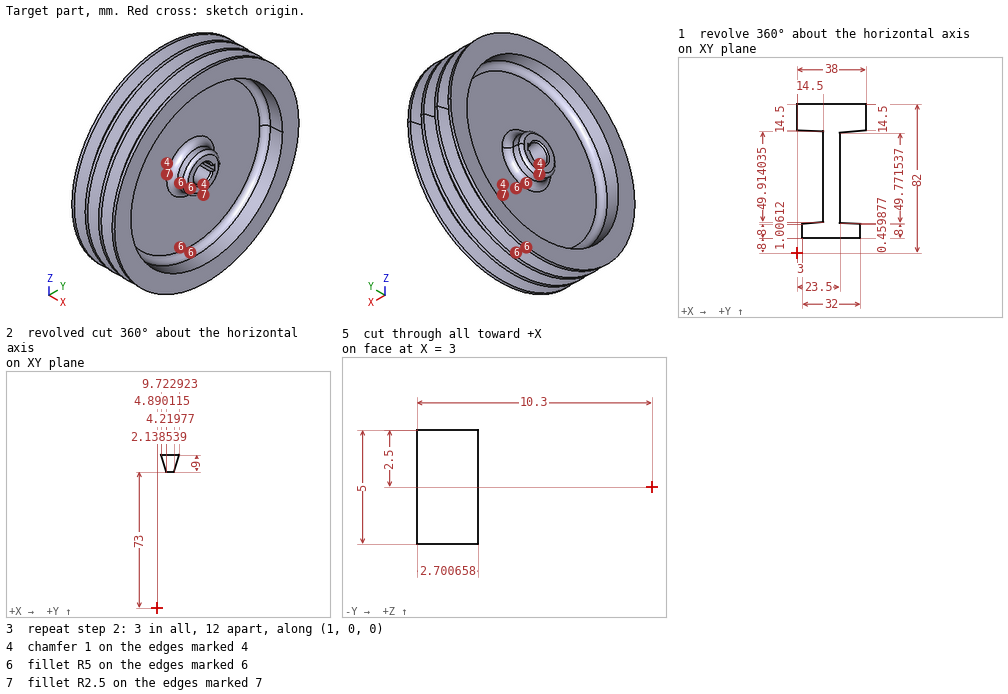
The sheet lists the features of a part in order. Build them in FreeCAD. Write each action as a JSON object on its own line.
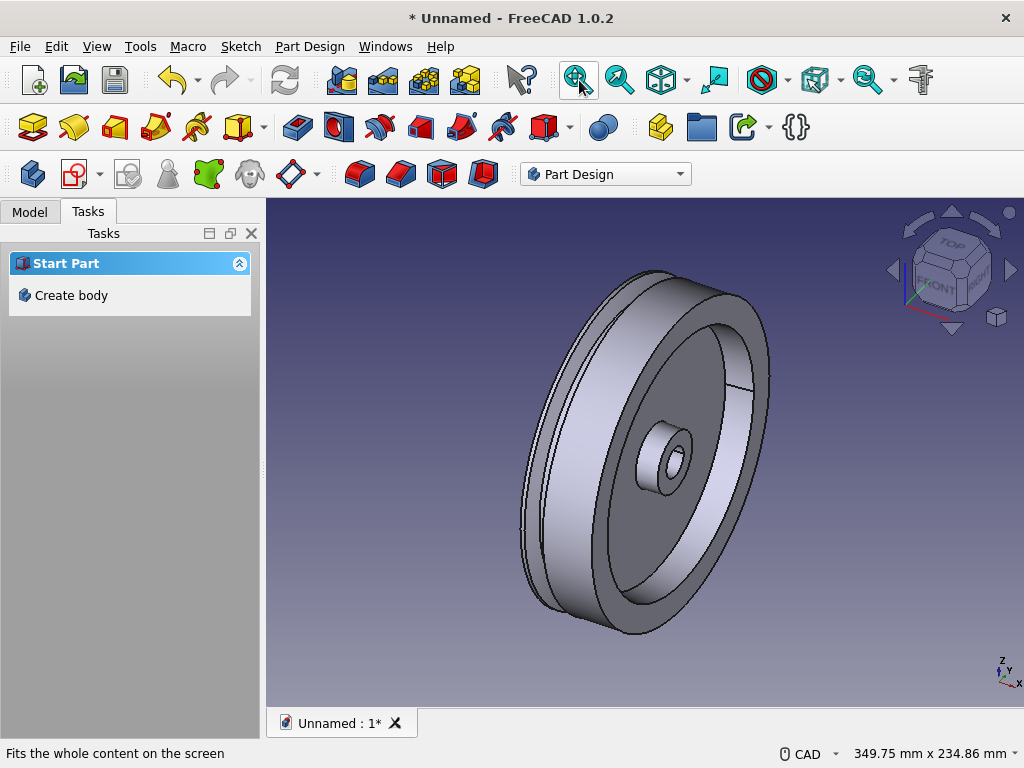
{"action": "left_click", "coordinate": [30, 212]}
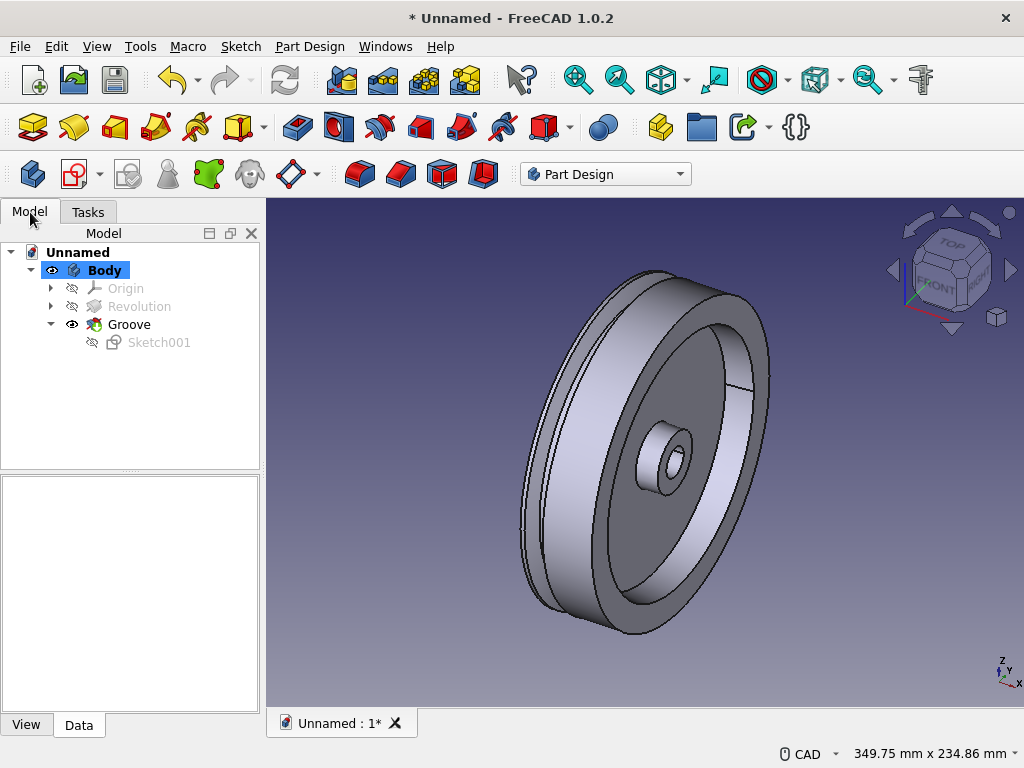
{"action": "left_click", "coordinate": [117, 324]}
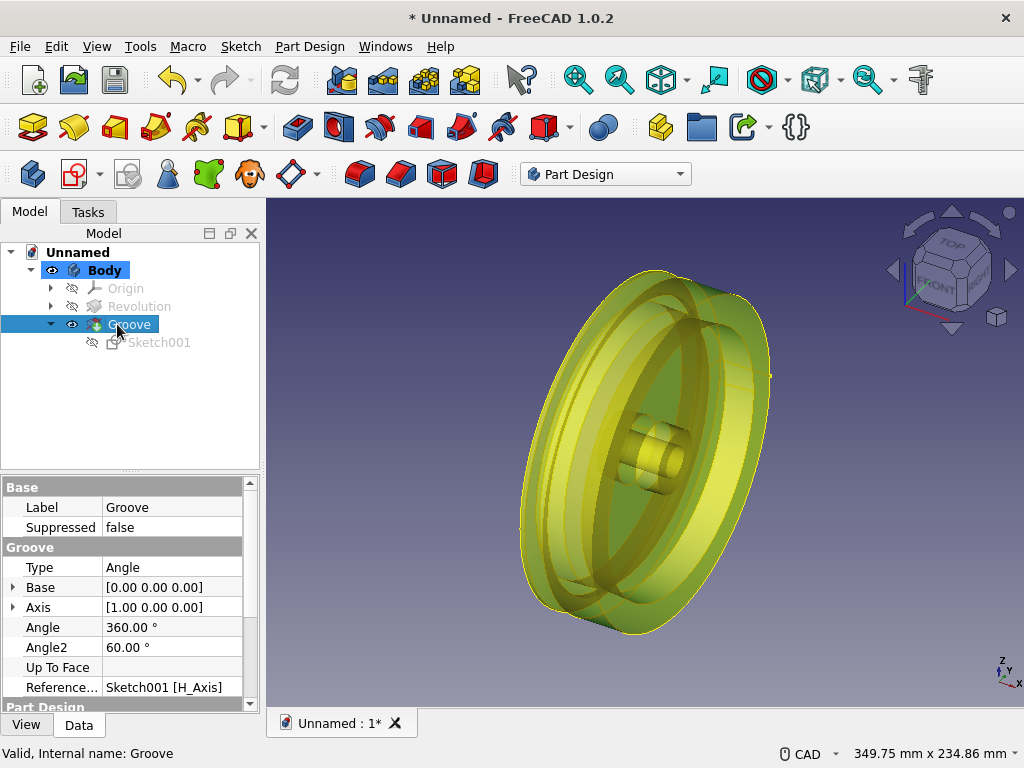
{"action": "left_click", "coordinate": [383, 80]}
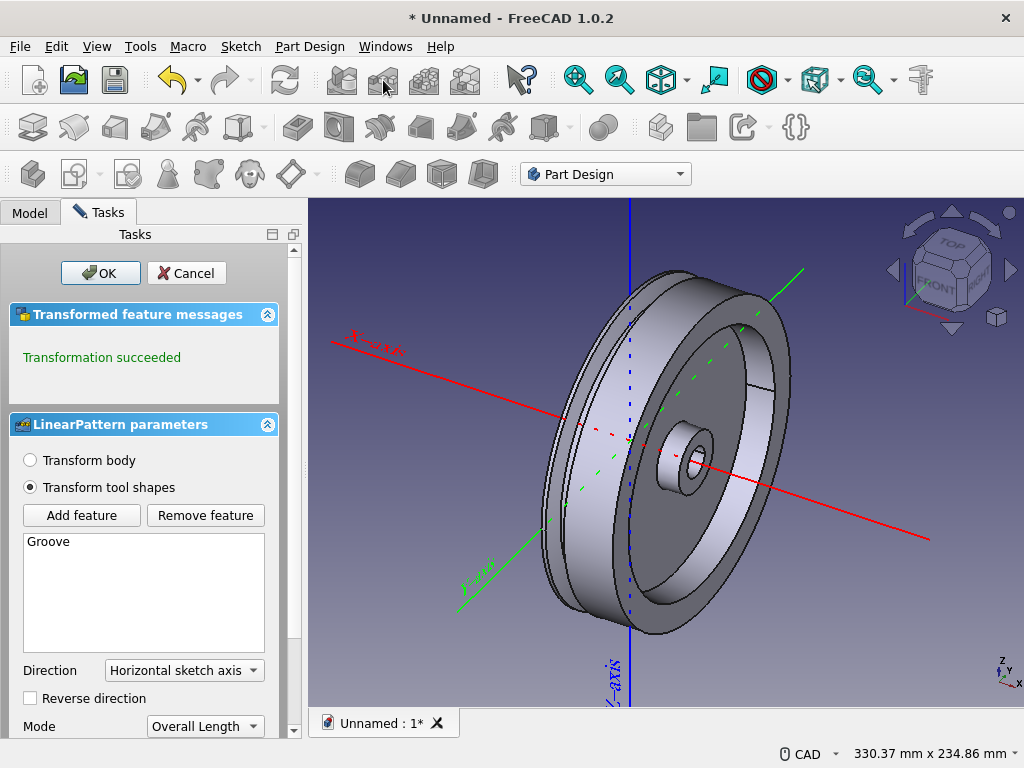
{"action": "left_click", "coordinate": [185, 670]}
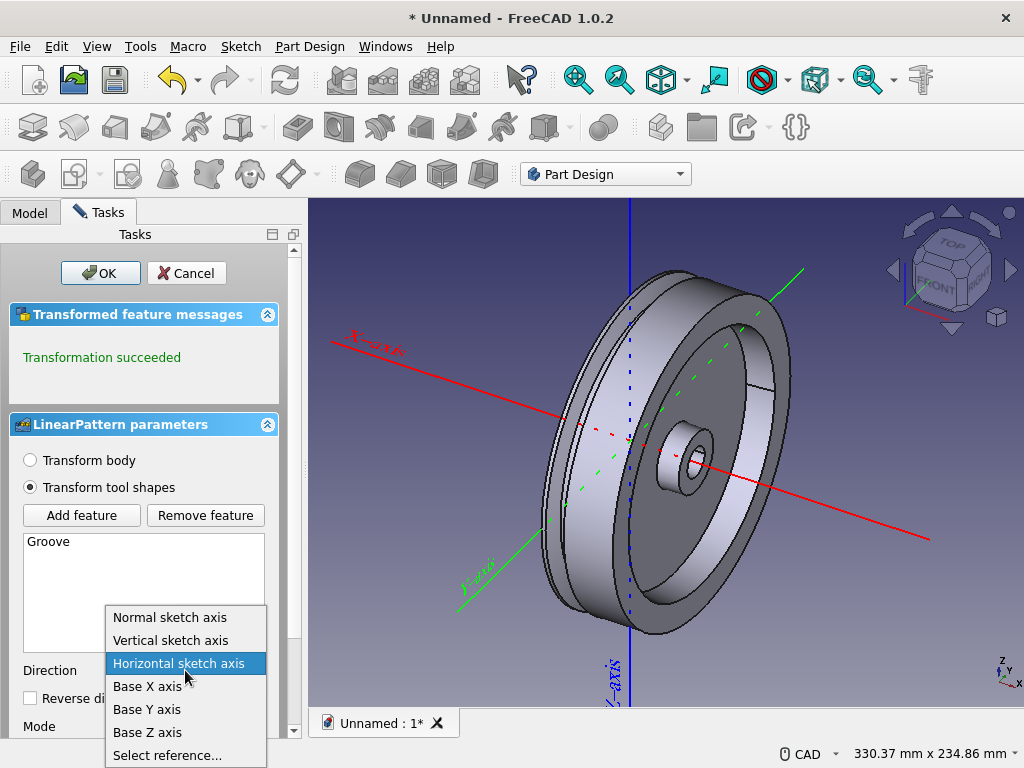
{"action": "left_click", "coordinate": [184, 686]}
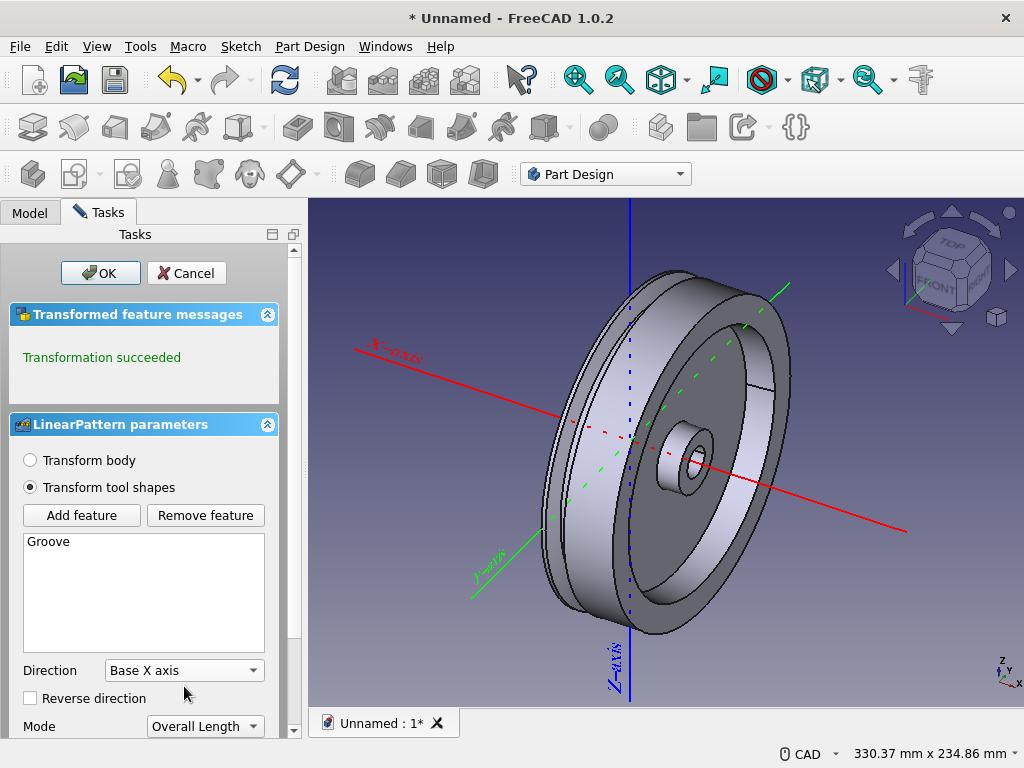
{"action": "left_click", "coordinate": [206, 726]}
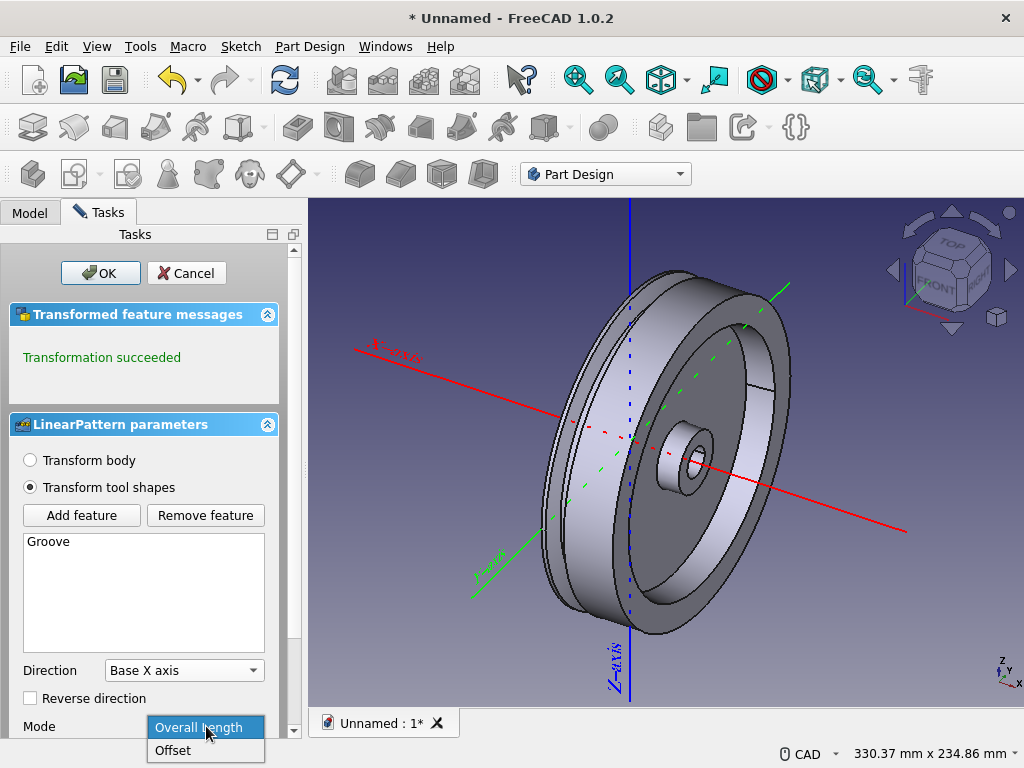
{"action": "left_click", "coordinate": [204, 750]}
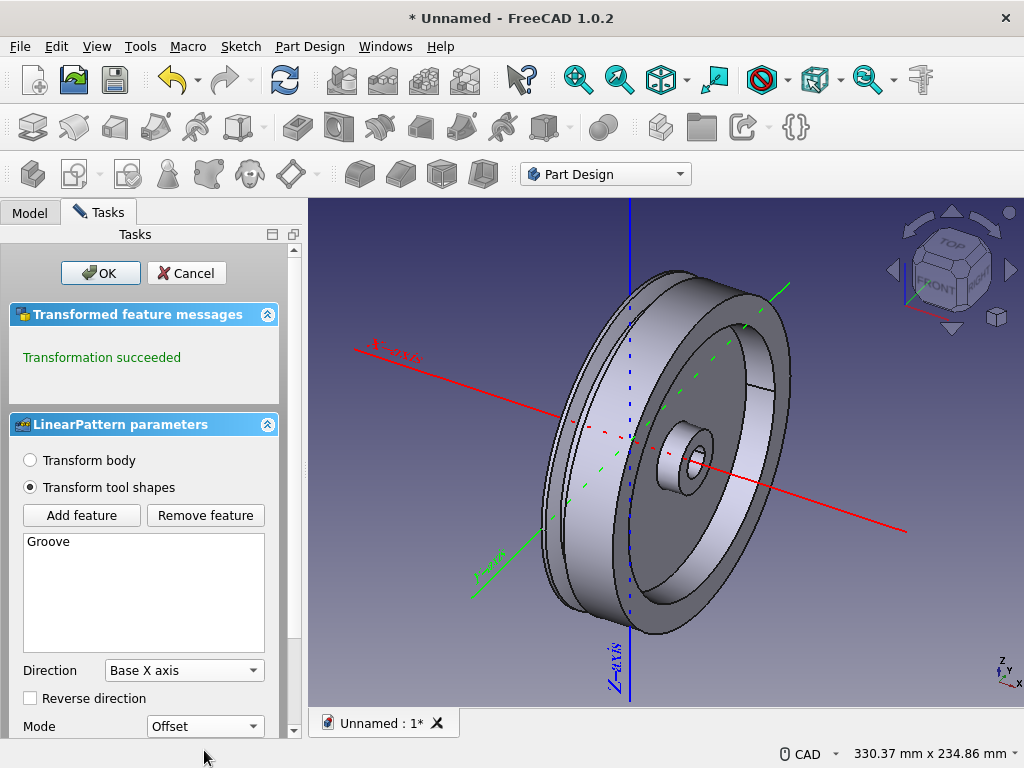
{"action": "scroll", "coordinate": [294, 491], "scroll_direction": "down", "scroll_amount": 2}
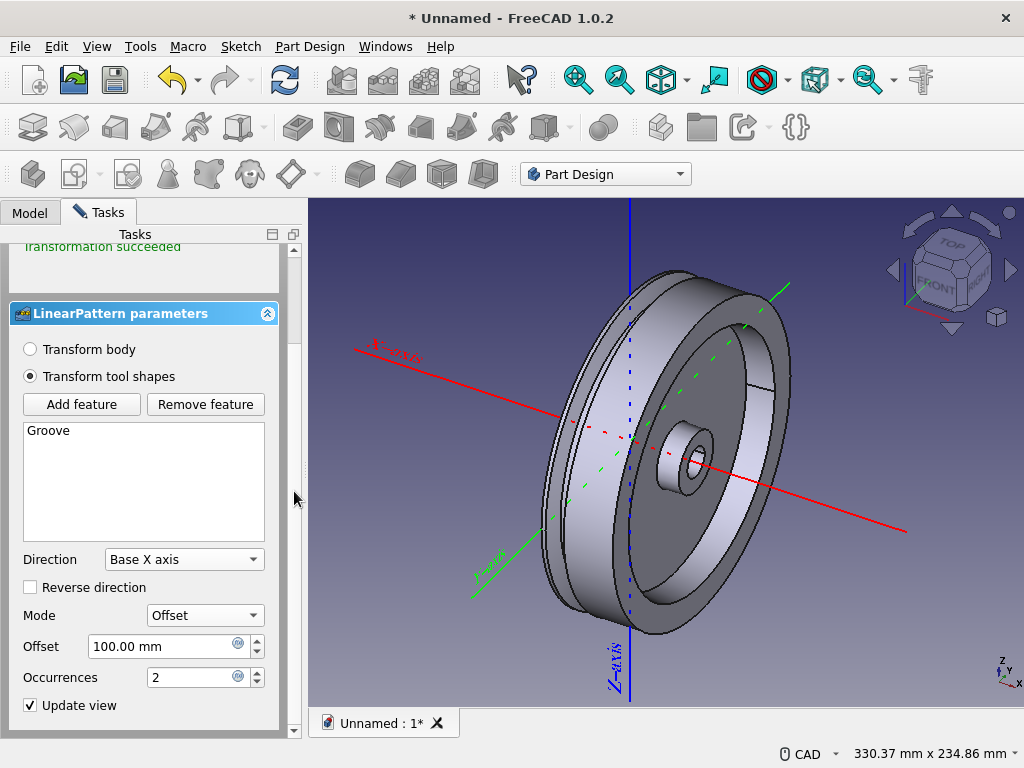
{"action": "triple_click", "coordinate": [170, 646]}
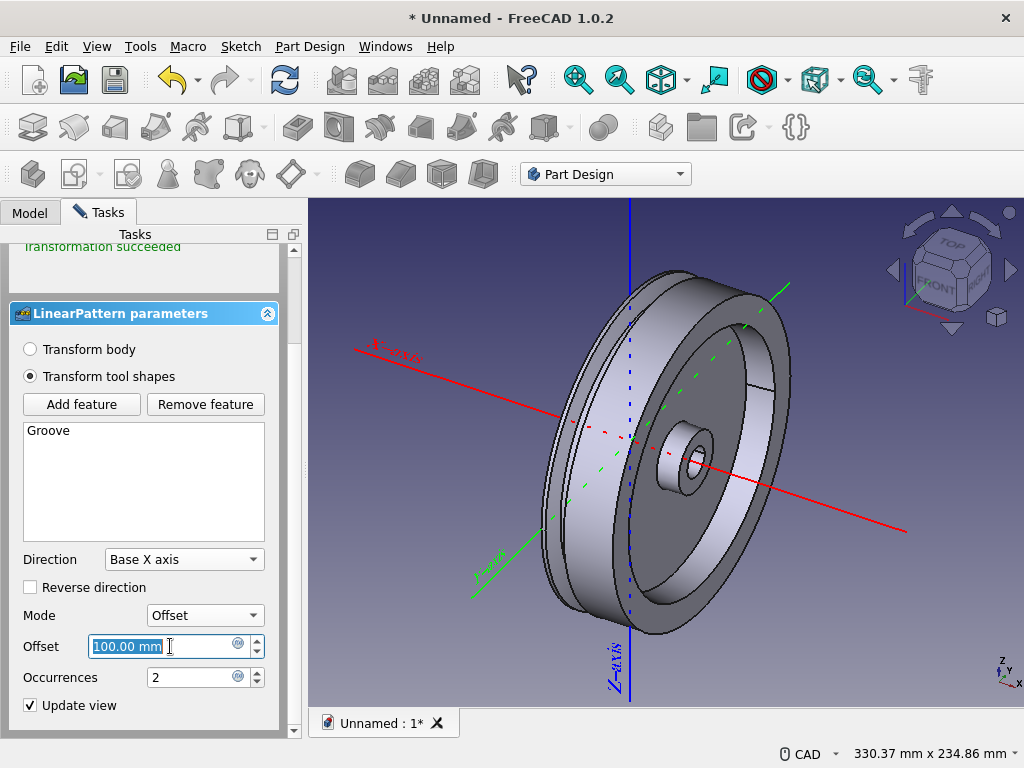
{"action": "type", "text": "12"}
{"action": "key", "text": "Tab"}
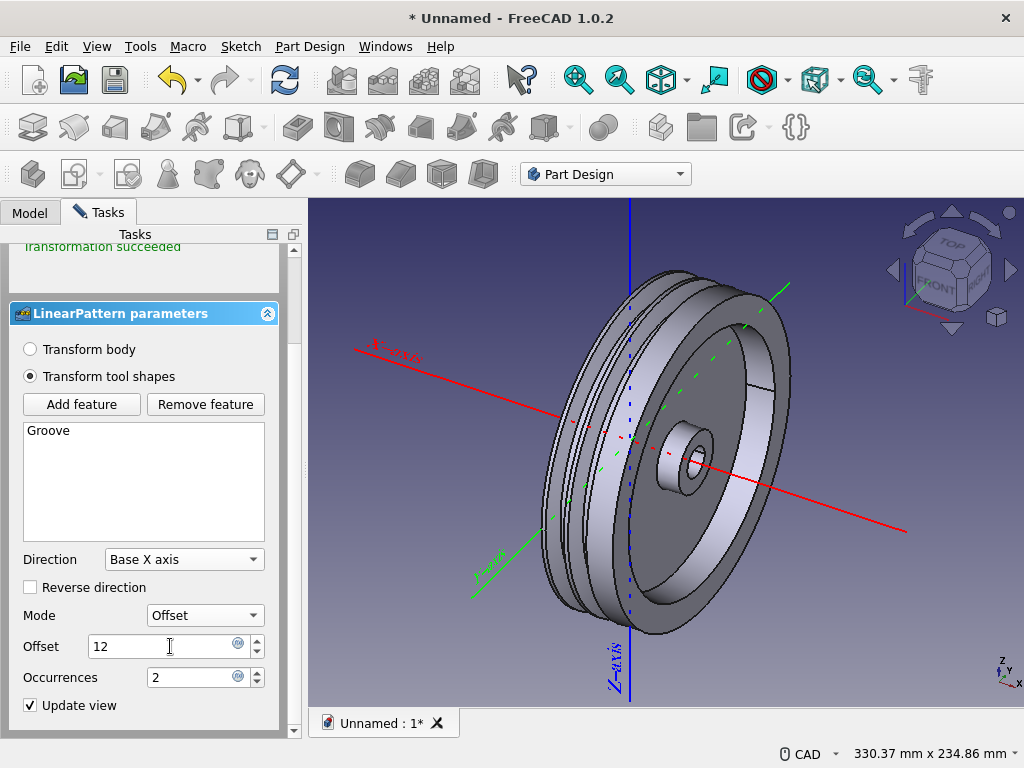
{"action": "triple_click", "coordinate": [199, 678]}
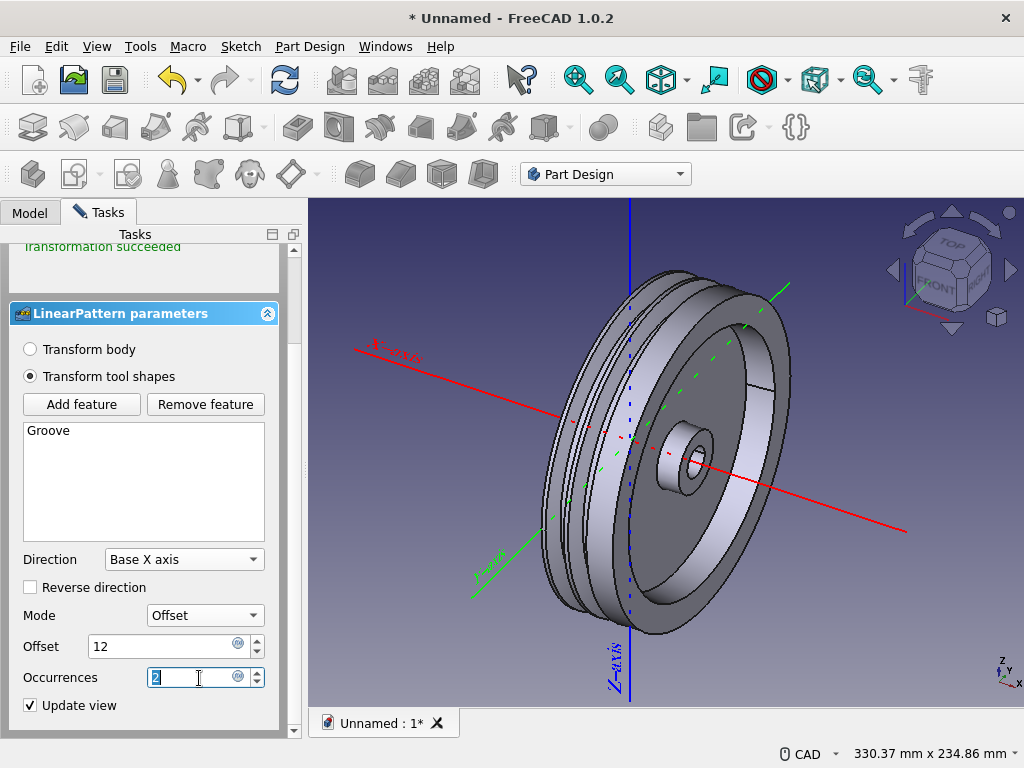
{"action": "type", "text": "3"}
{"action": "key", "text": "Tab"}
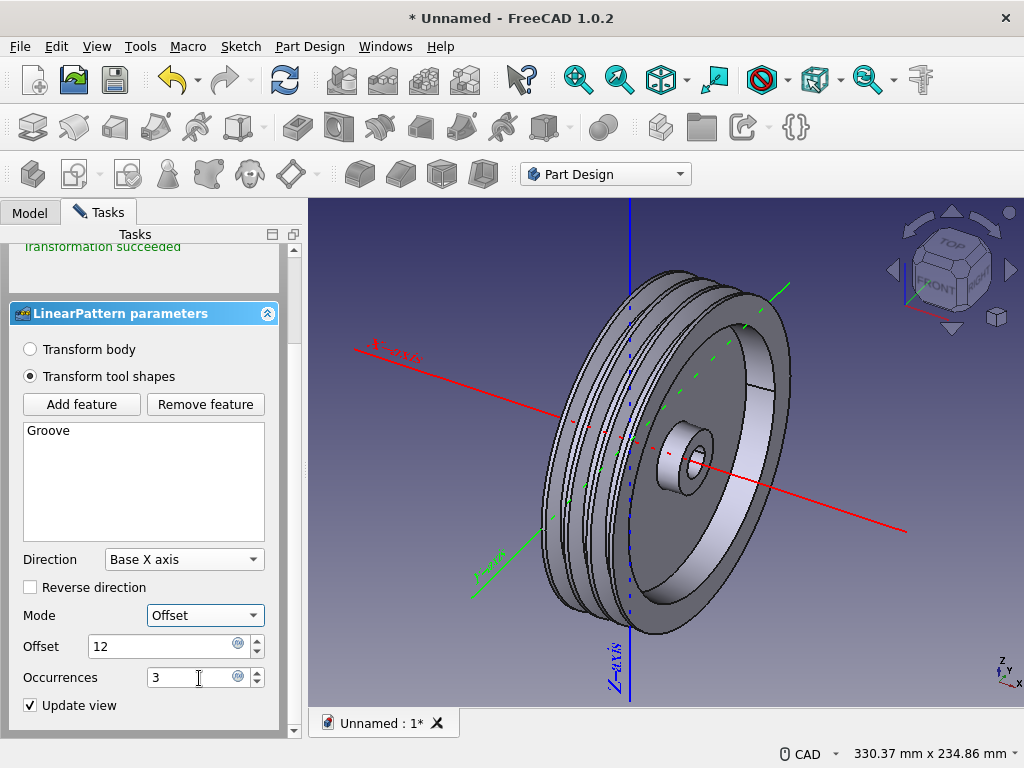
{"action": "scroll", "coordinate": [294, 491], "scroll_direction": "up", "scroll_amount": 3}